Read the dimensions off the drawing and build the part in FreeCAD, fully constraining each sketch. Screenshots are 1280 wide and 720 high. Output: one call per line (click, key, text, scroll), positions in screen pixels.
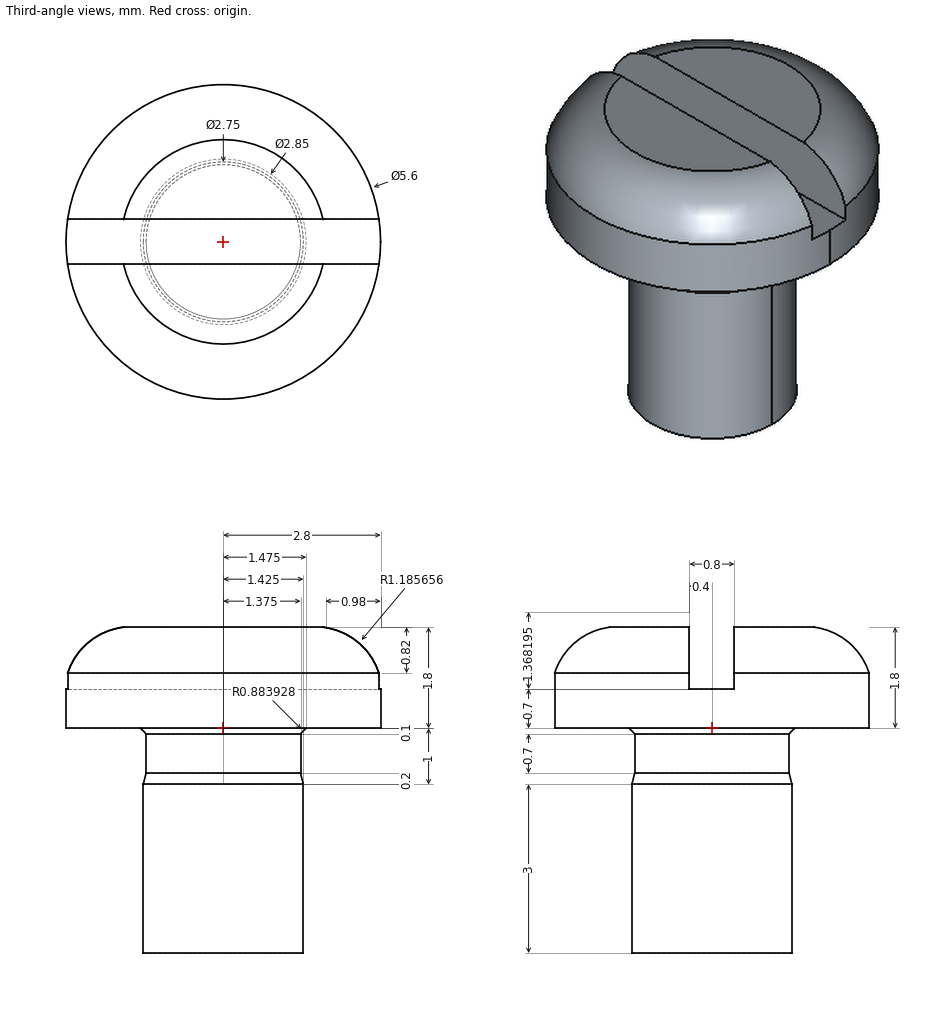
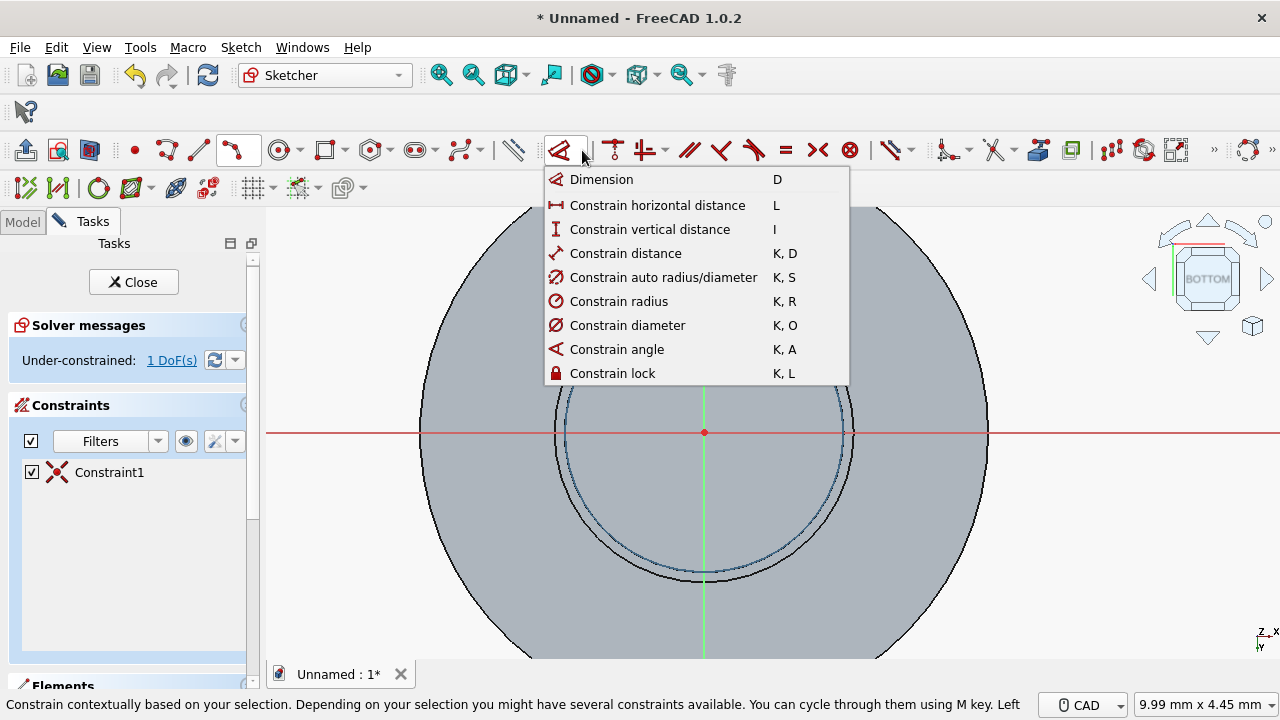
click(697, 325)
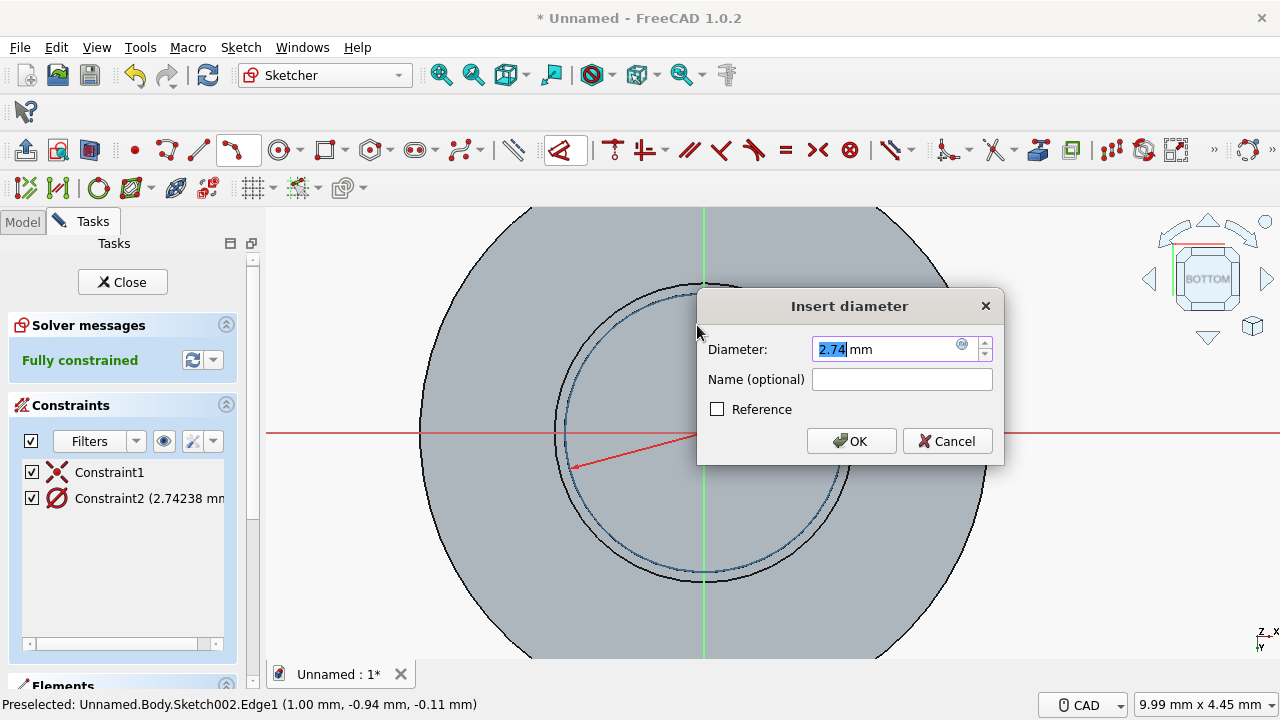
text(2.75)
key(Return)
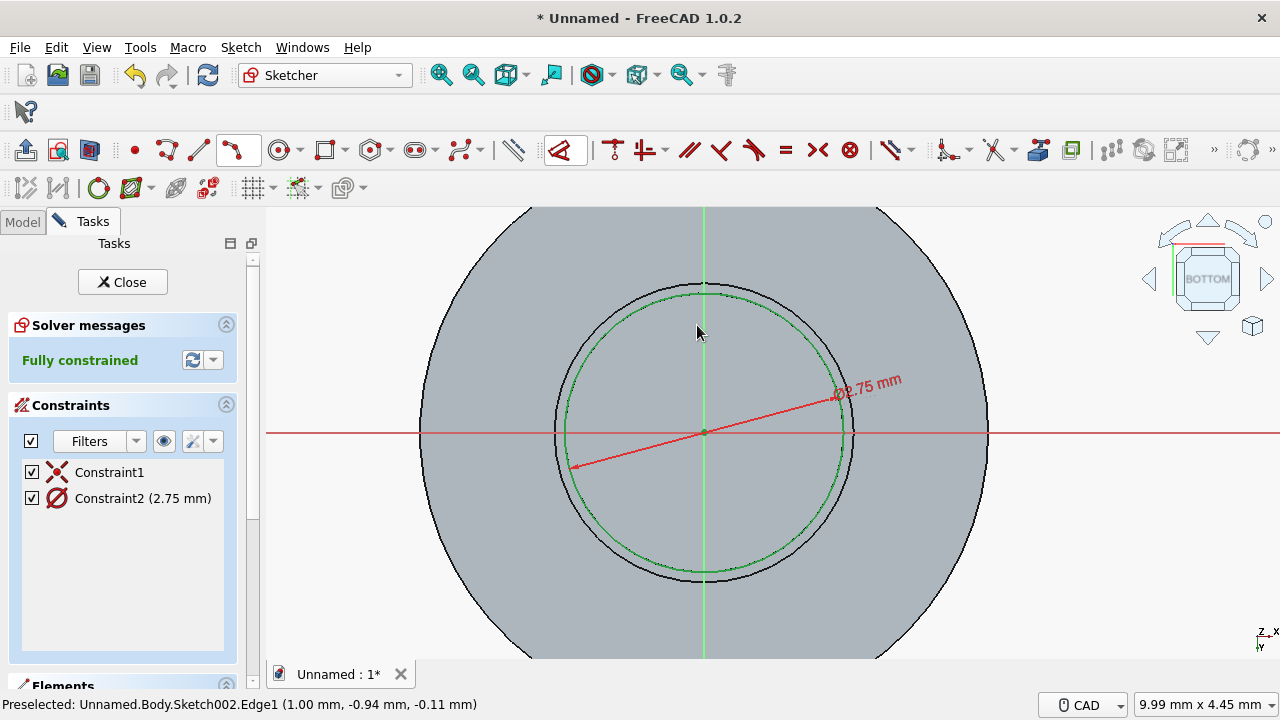
click(123, 282)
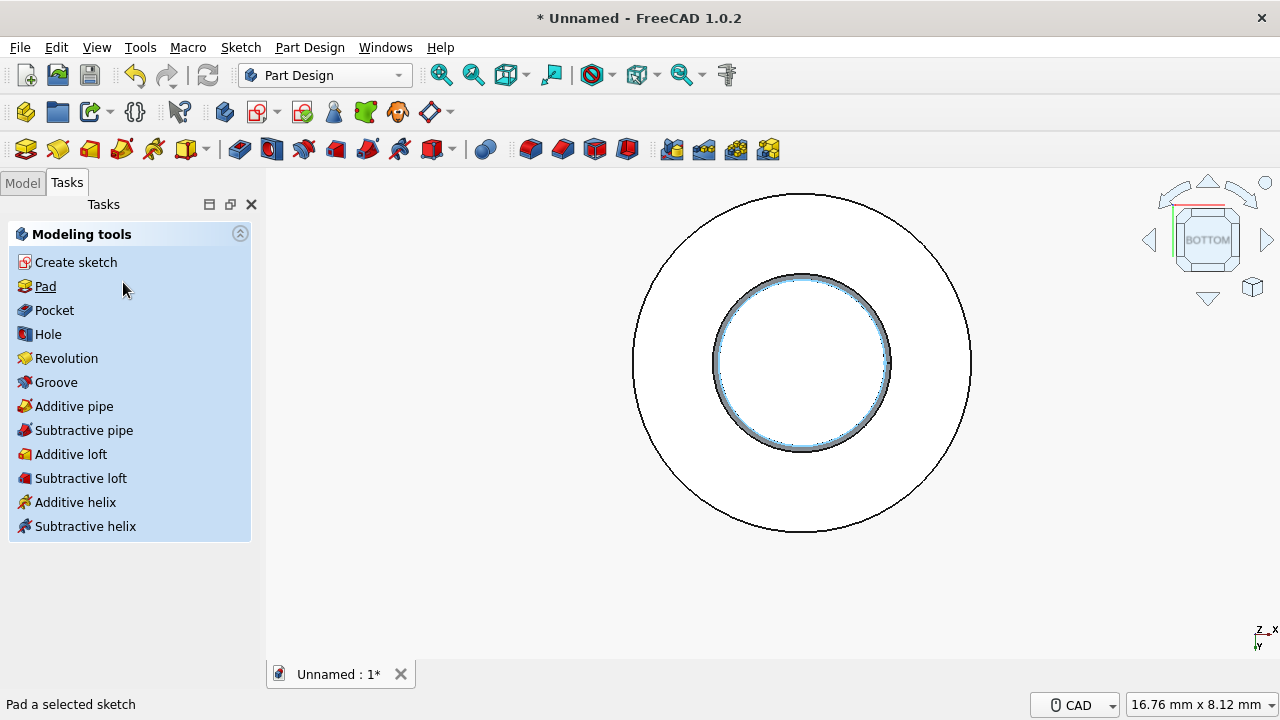
click(26, 150)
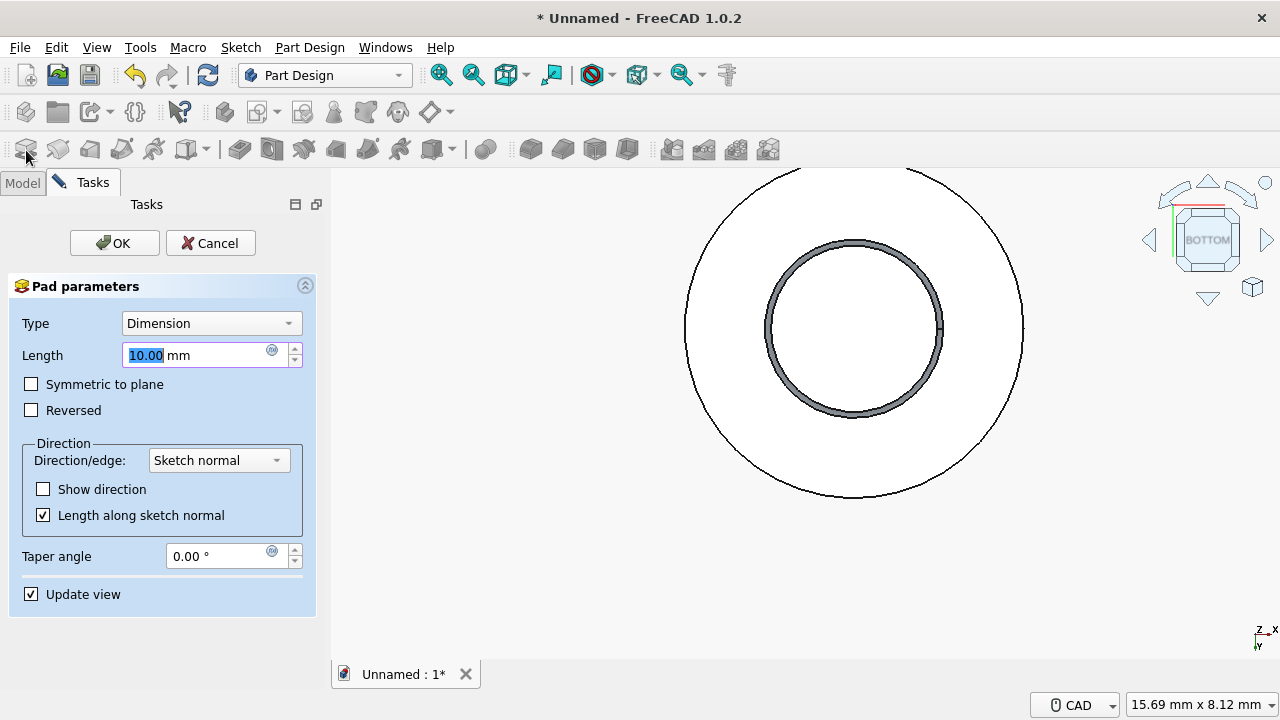
text(0.7)
key(Tab)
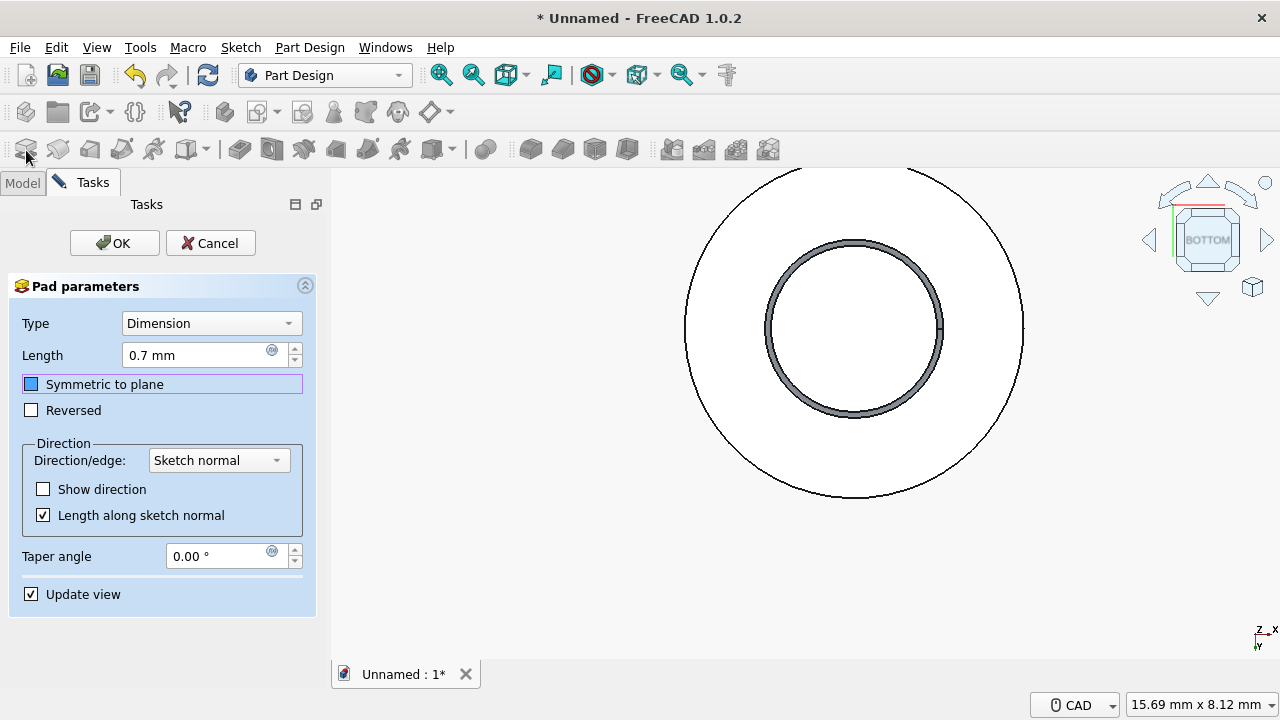
click(115, 243)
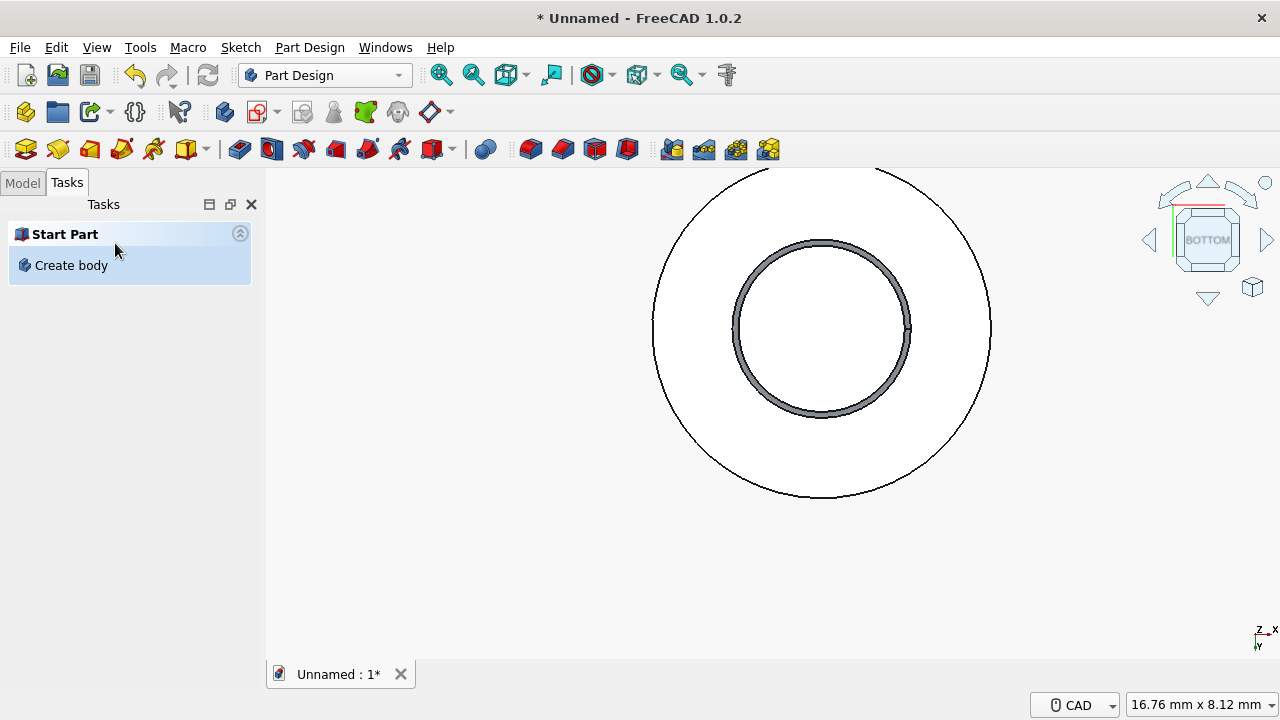
click(442, 76)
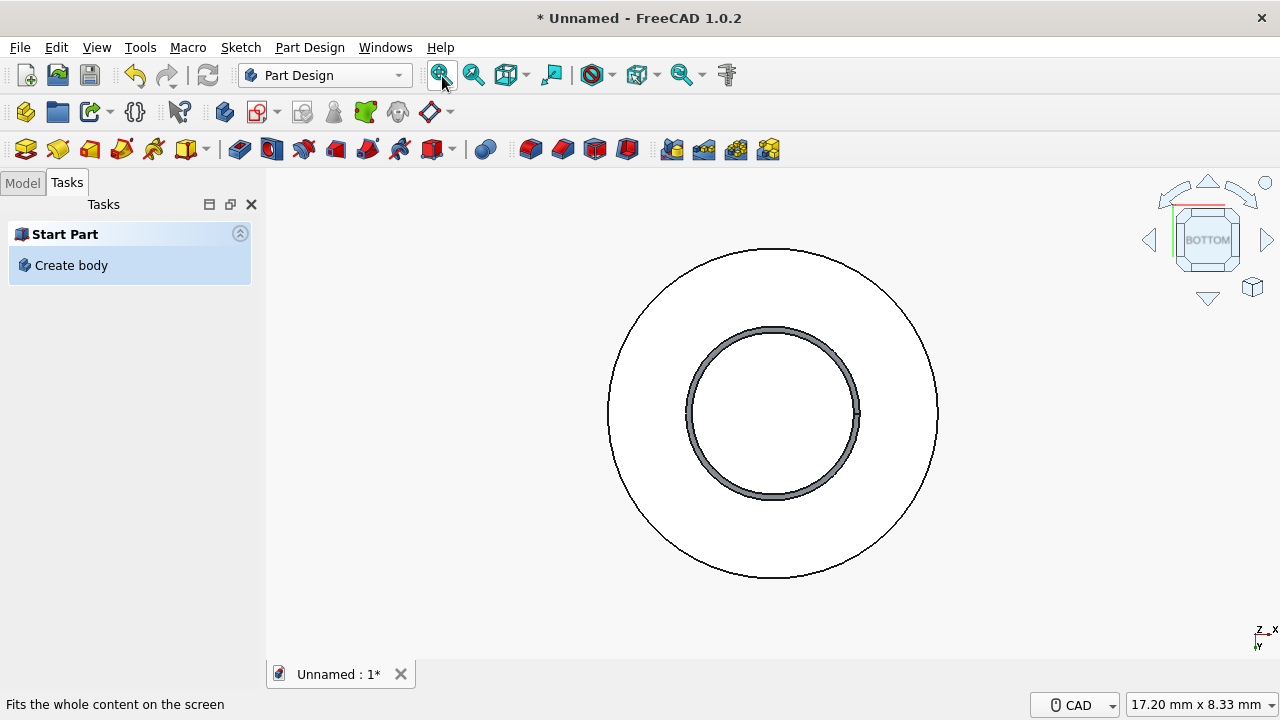
click(258, 112)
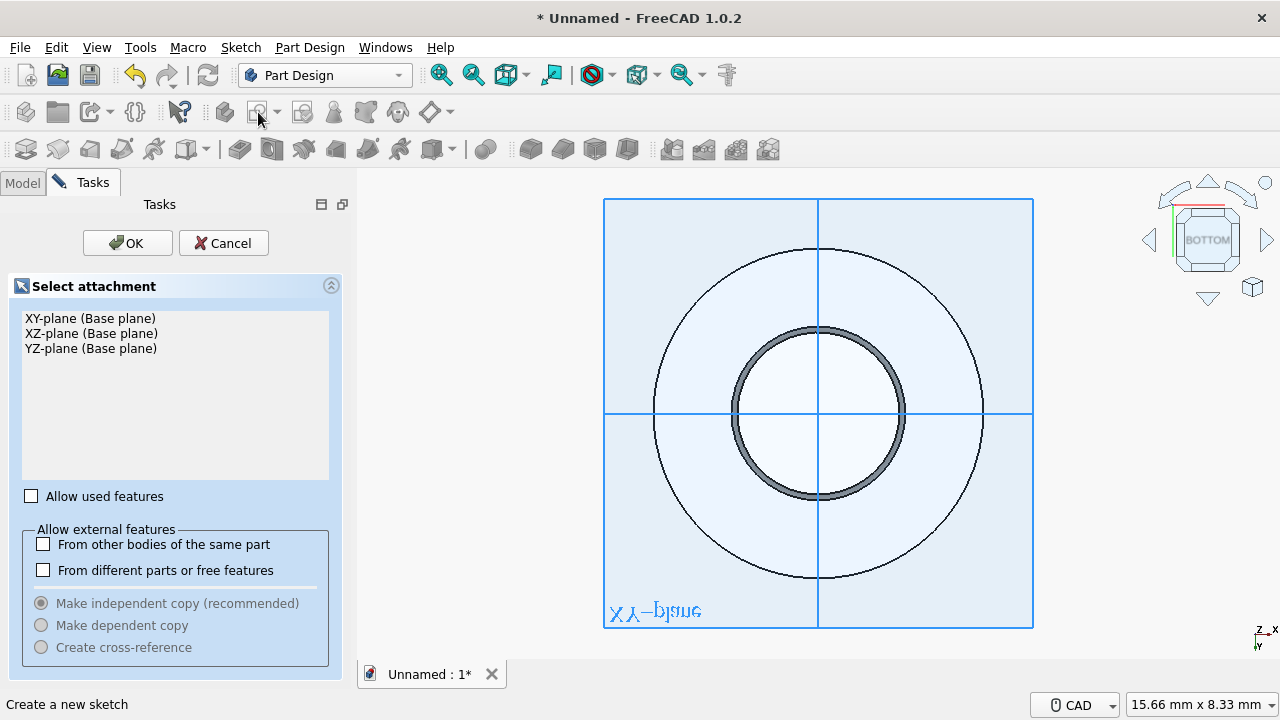
click(82, 334)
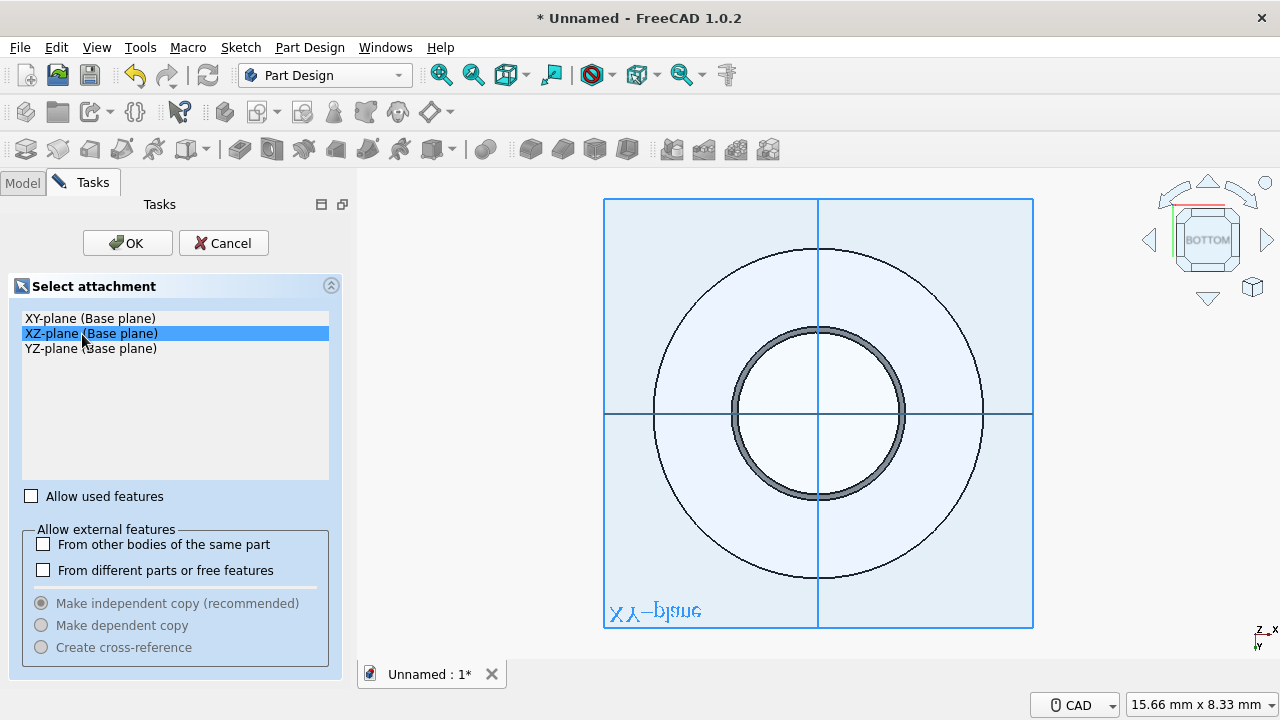
click(128, 243)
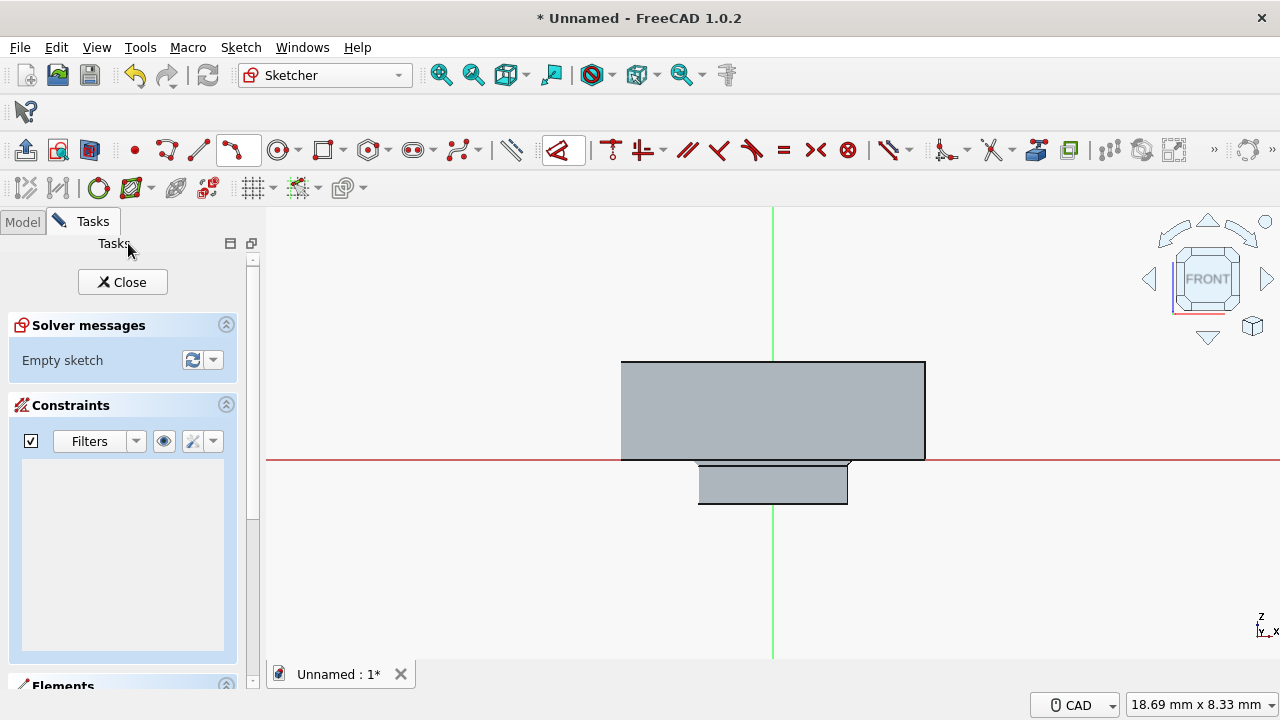
click(90, 150)